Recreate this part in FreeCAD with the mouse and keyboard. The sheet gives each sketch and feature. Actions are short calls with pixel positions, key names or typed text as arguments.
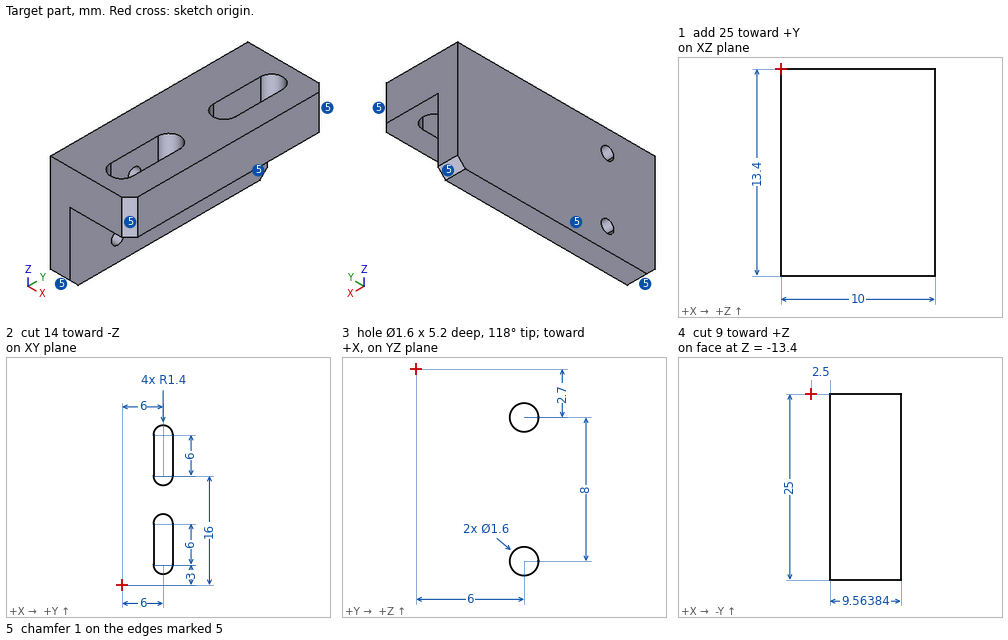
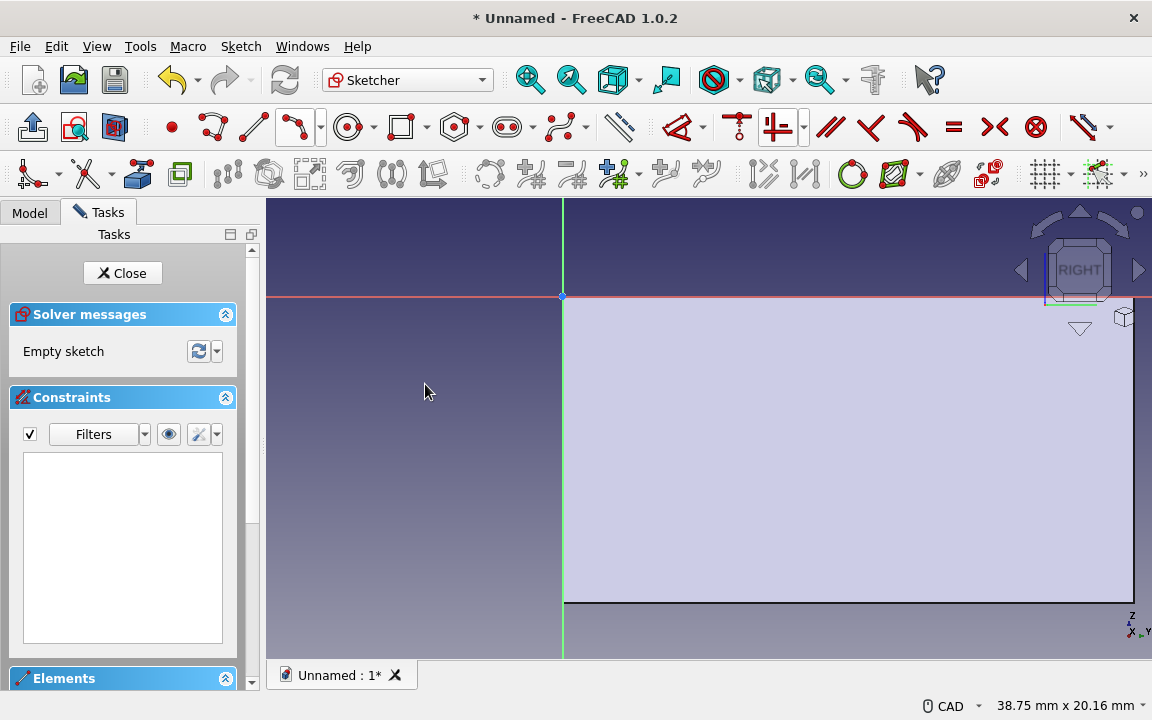
key(g)
key(c)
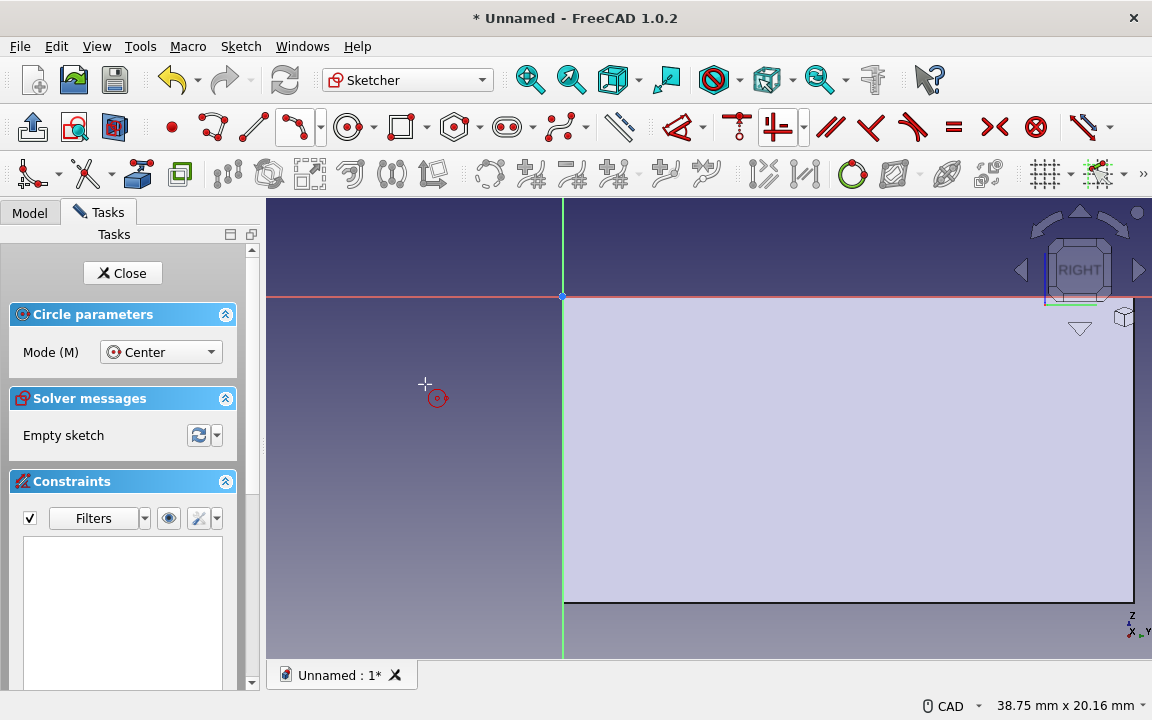
scroll(700, 542, up, 2)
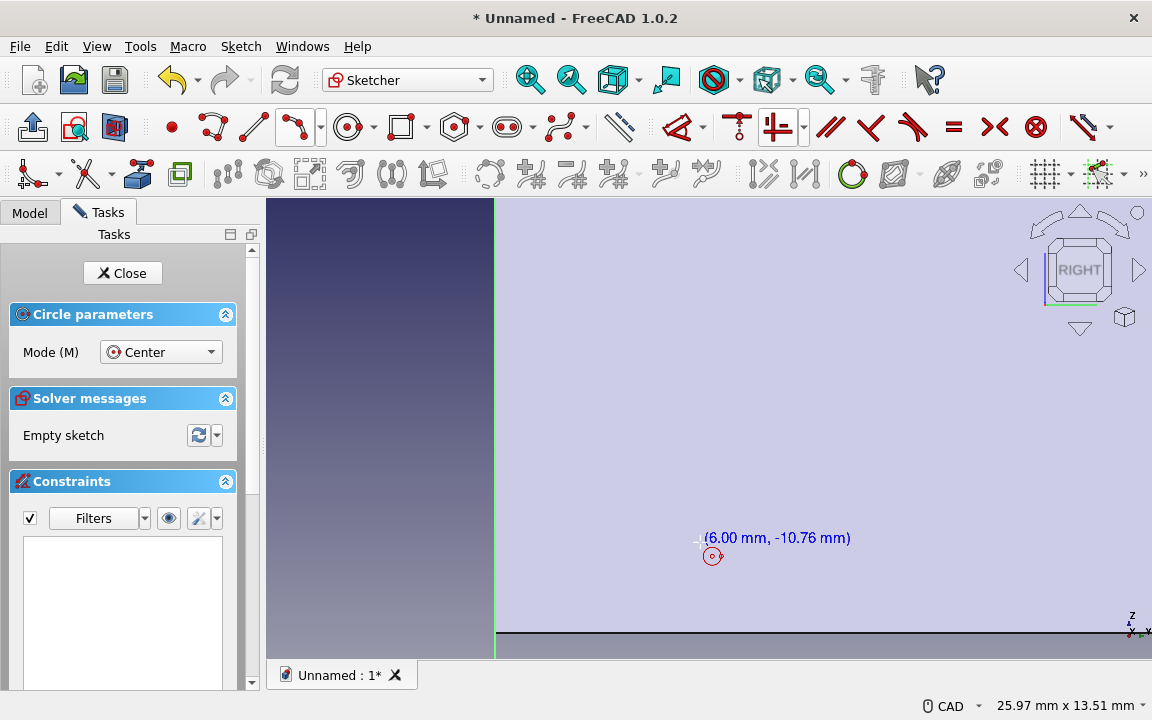
click(700, 541)
click(719, 522)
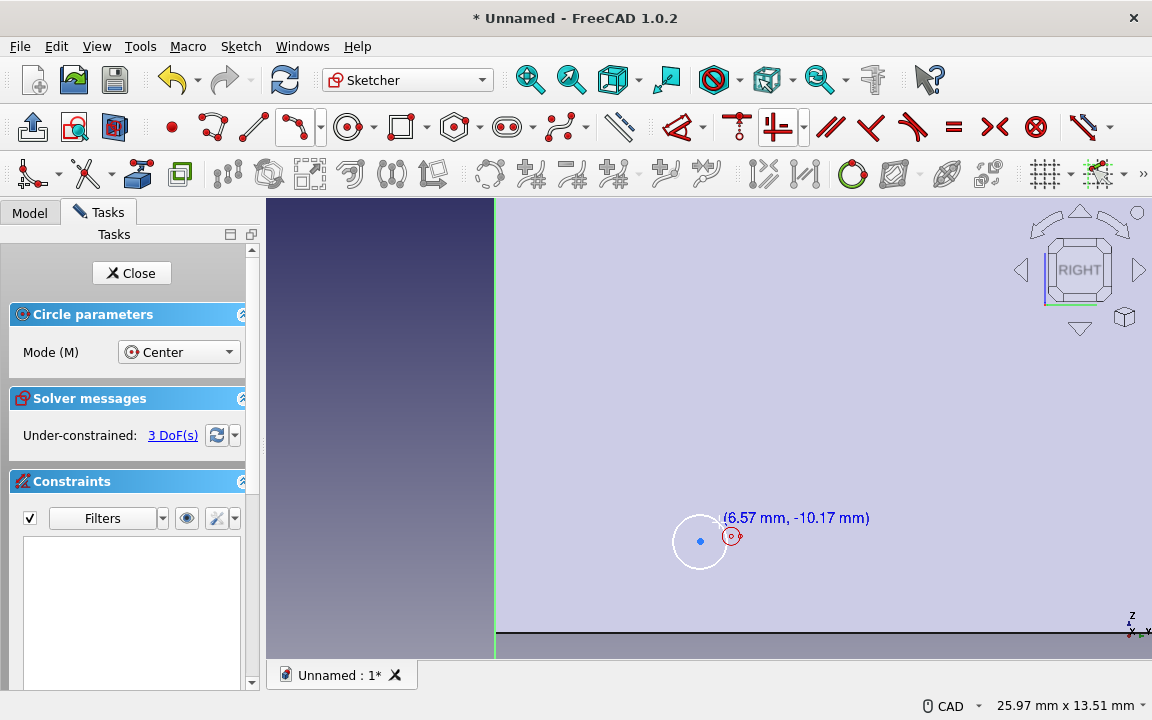
click(700, 268)
click(719, 249)
key(Escape)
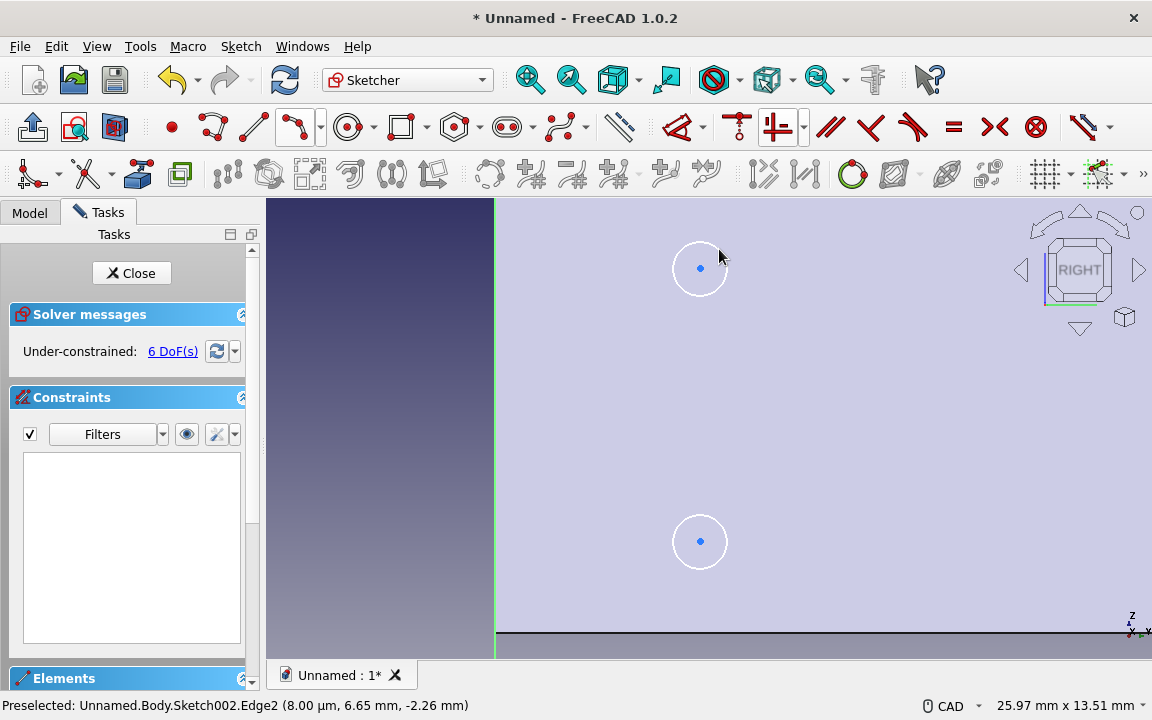
click(719, 523)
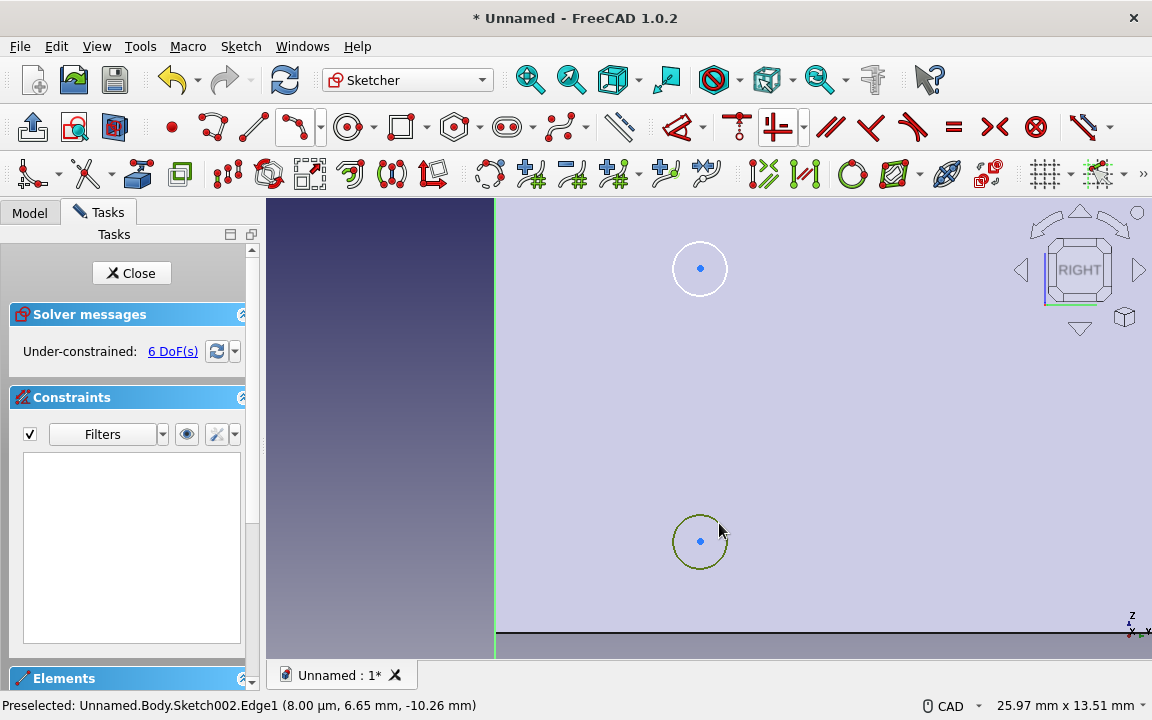
click(719, 250)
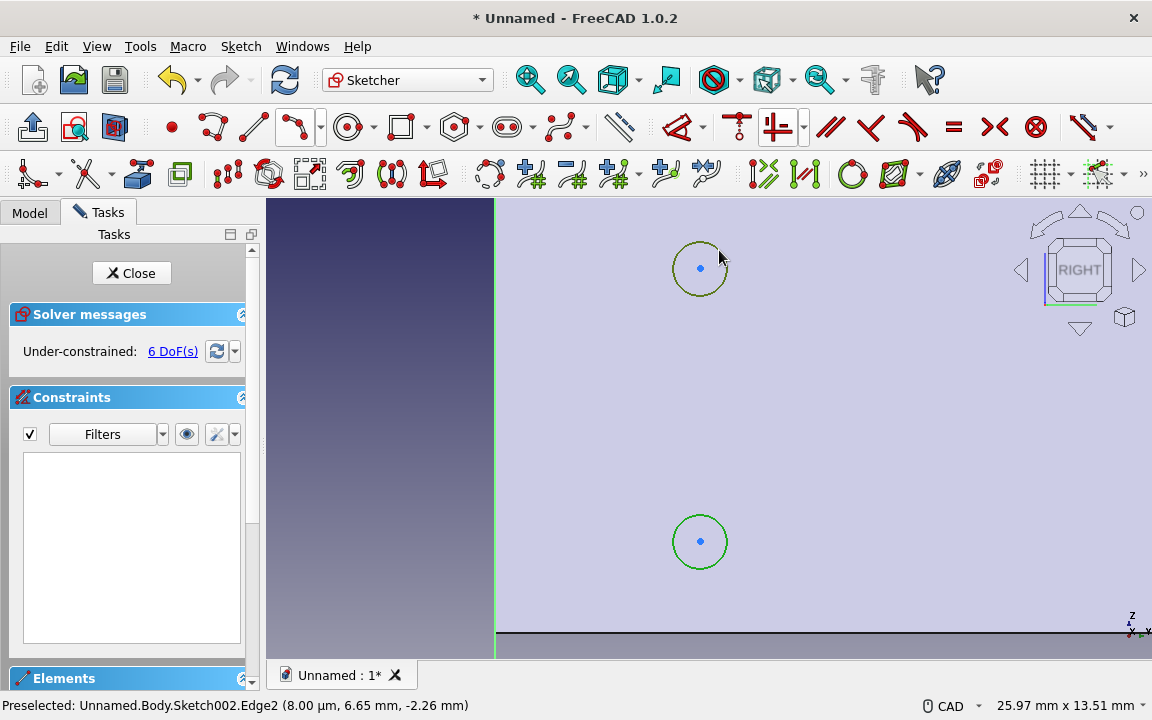
click(954, 128)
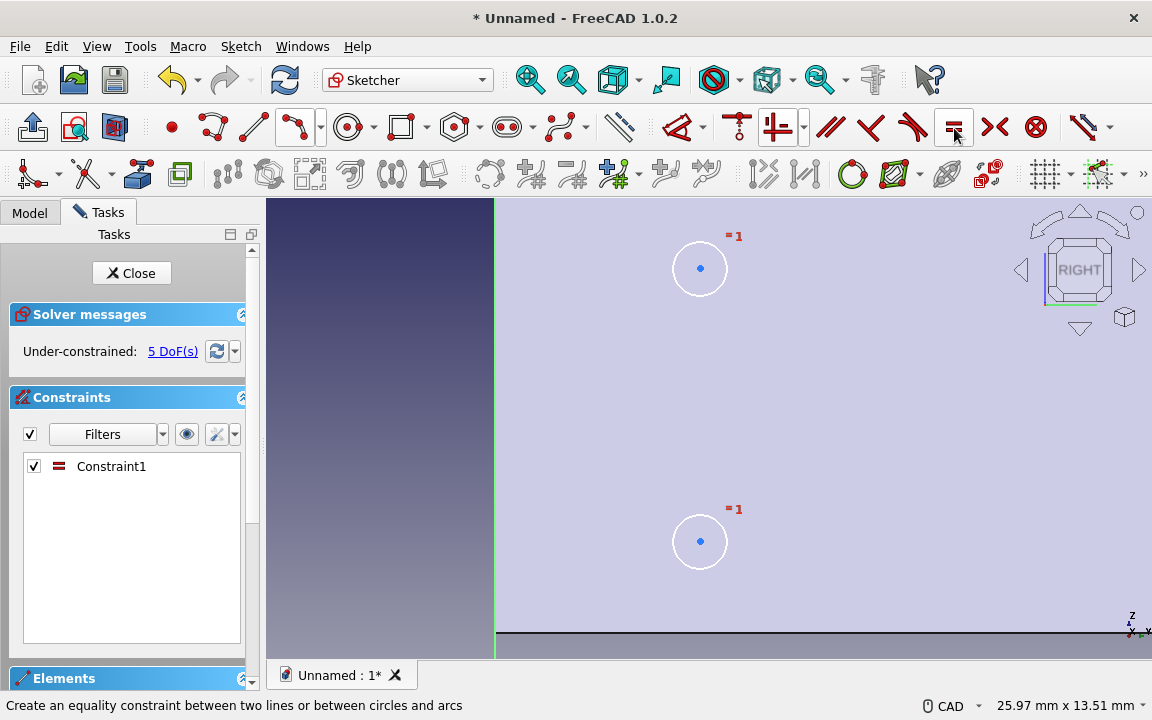
click(700, 542)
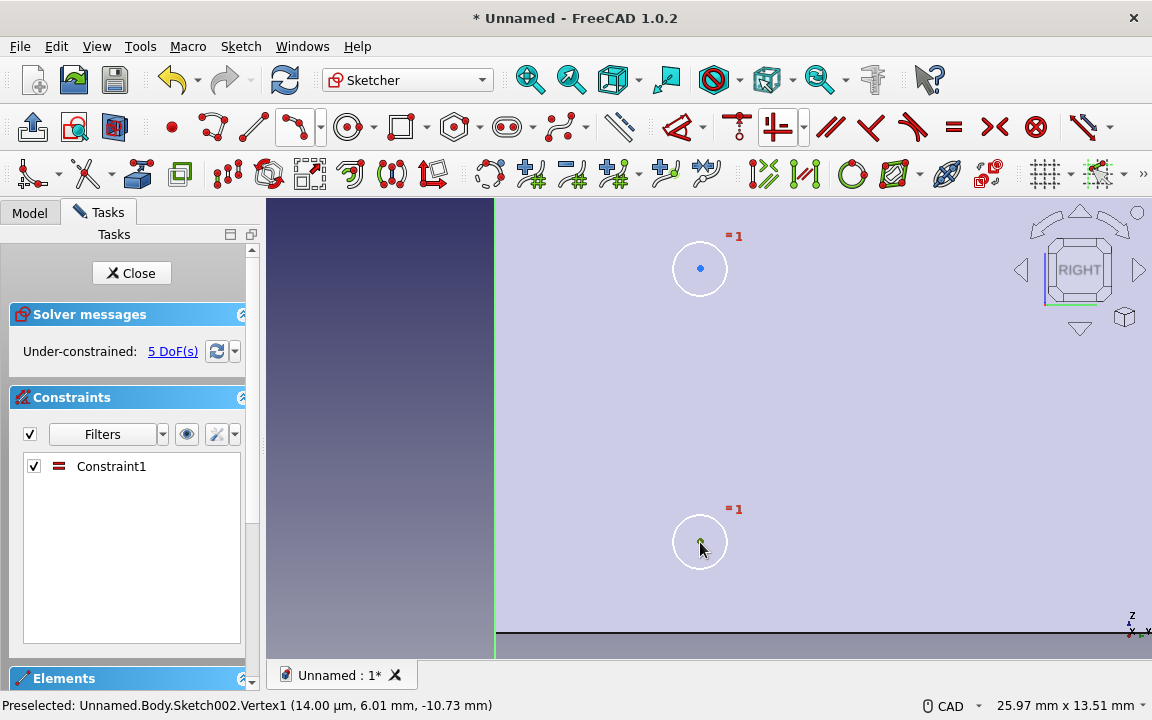
click(700, 269)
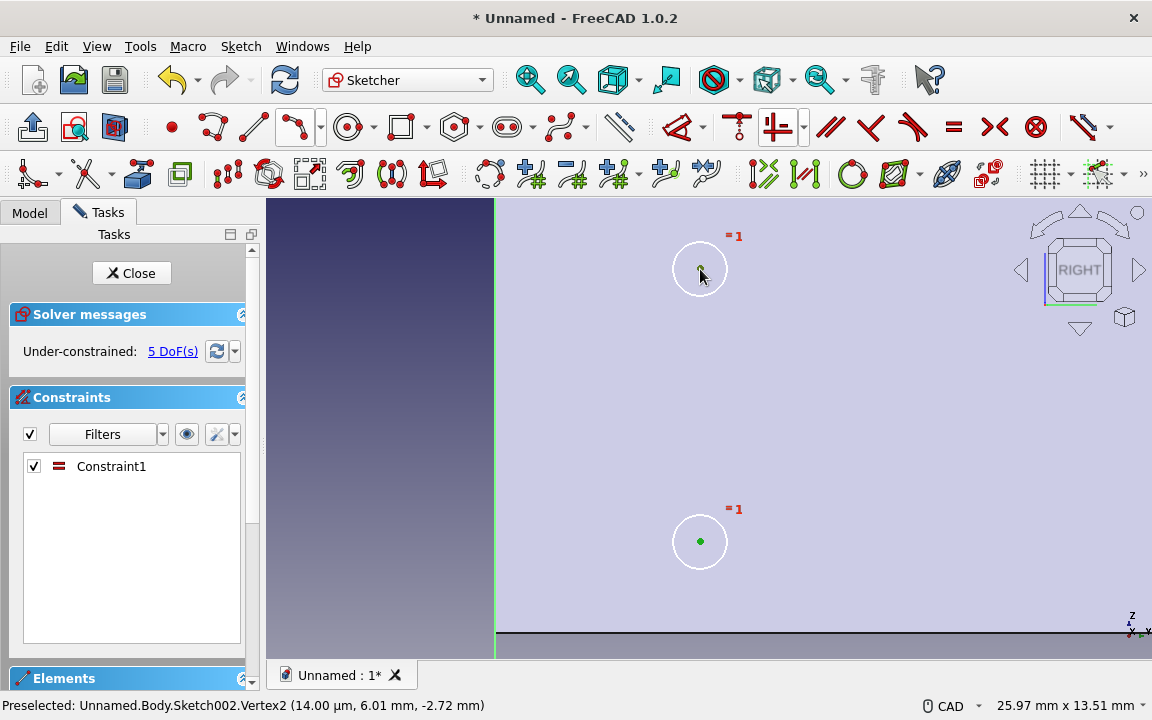
click(804, 128)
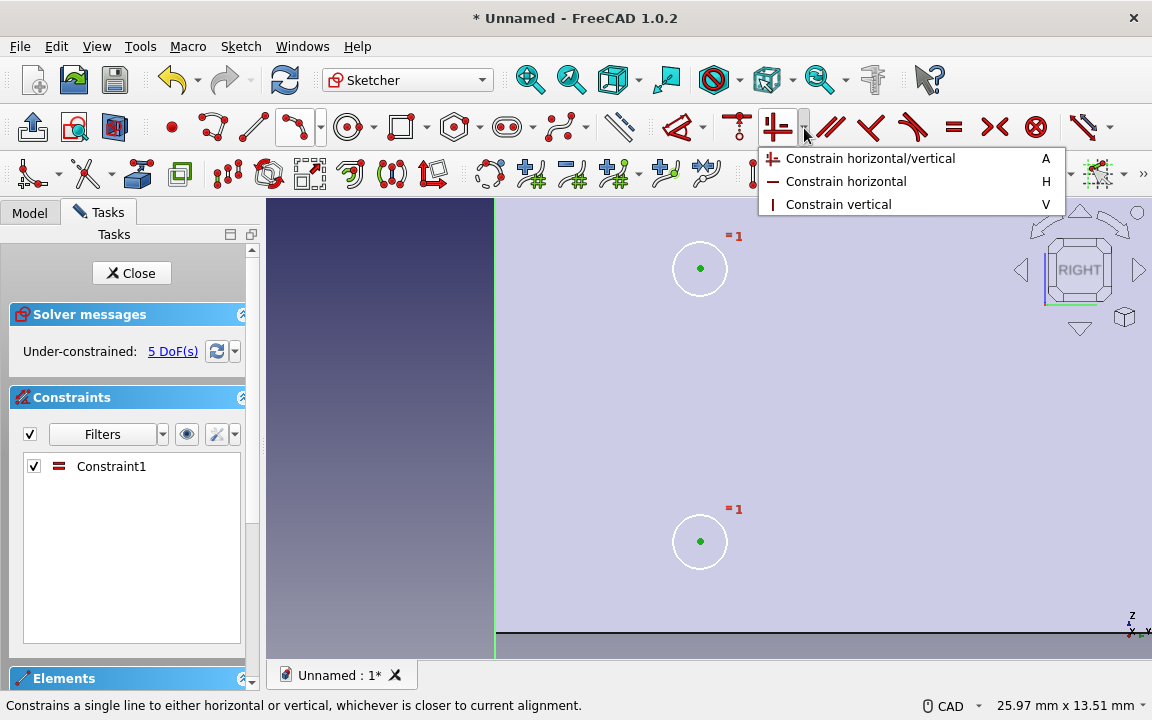
click(912, 204)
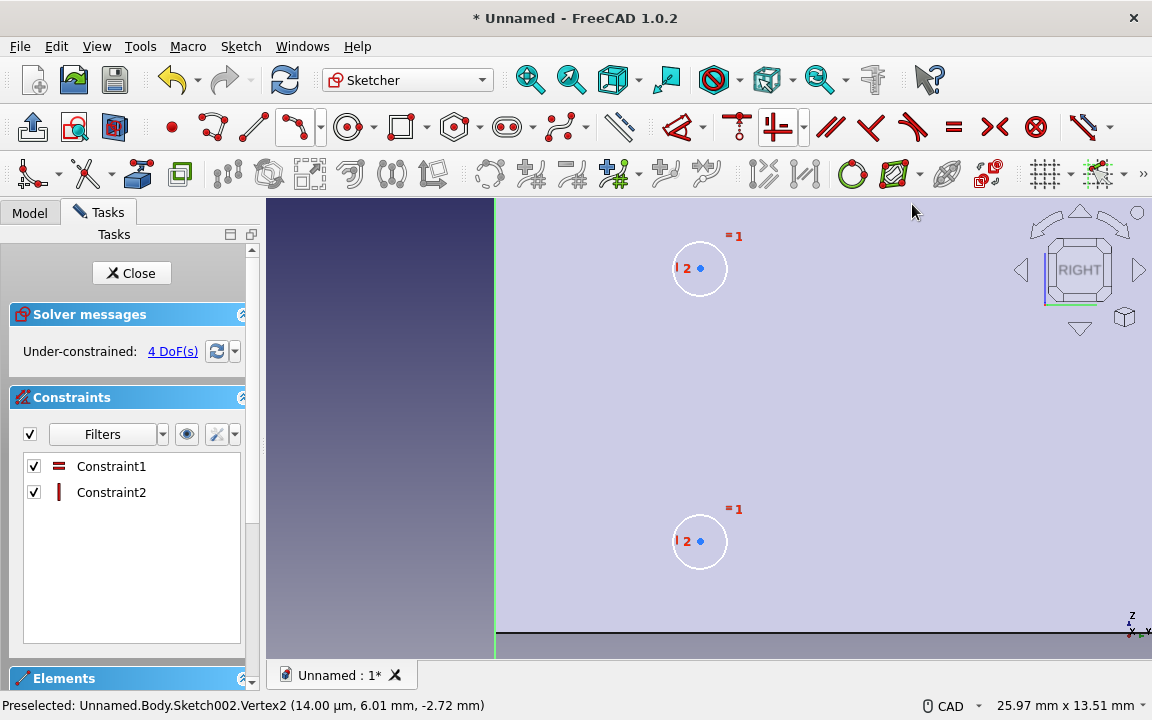
click(676, 128)